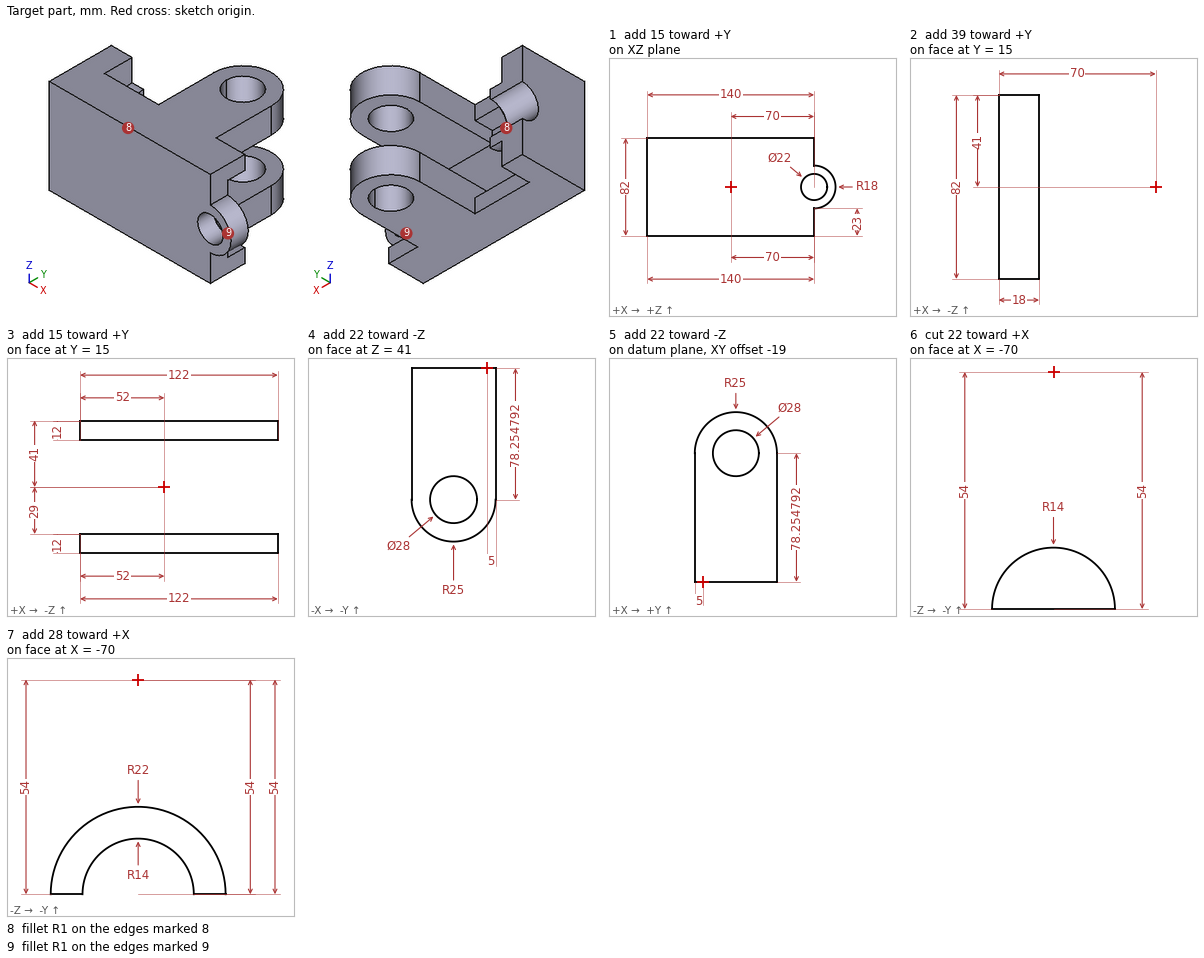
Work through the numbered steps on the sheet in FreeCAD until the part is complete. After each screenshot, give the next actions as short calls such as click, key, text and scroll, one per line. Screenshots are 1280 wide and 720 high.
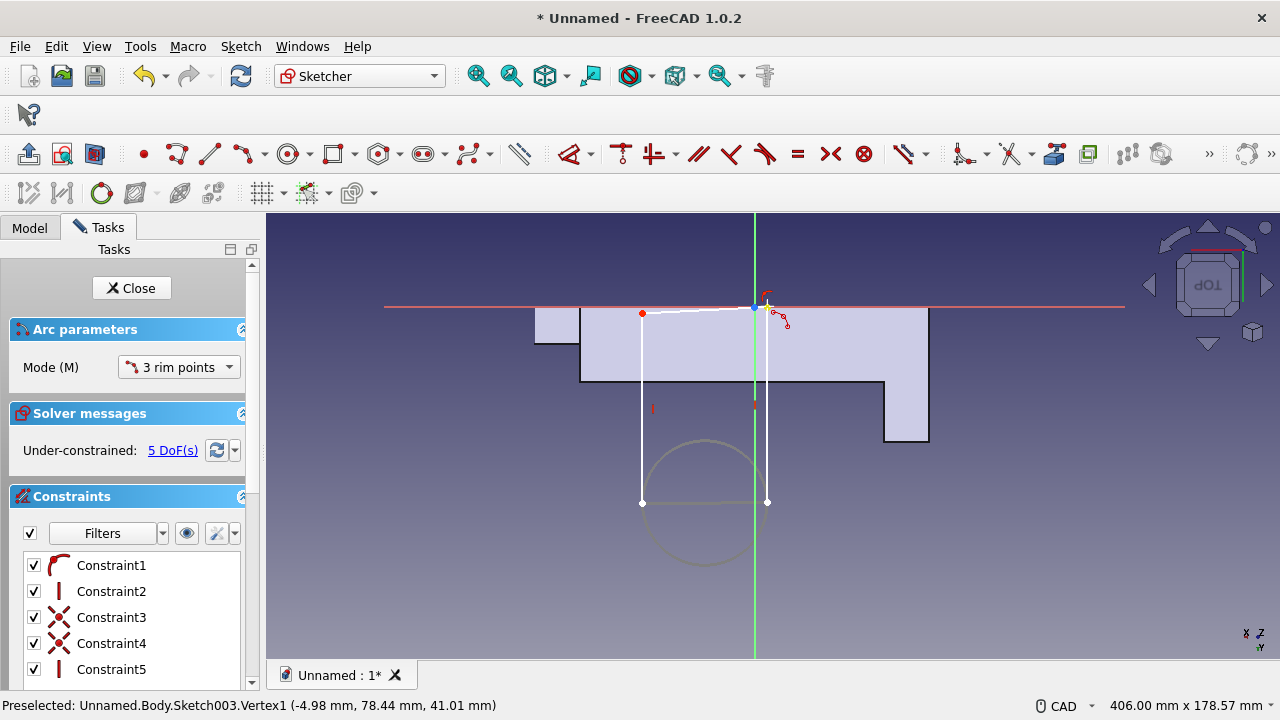
click(705, 565)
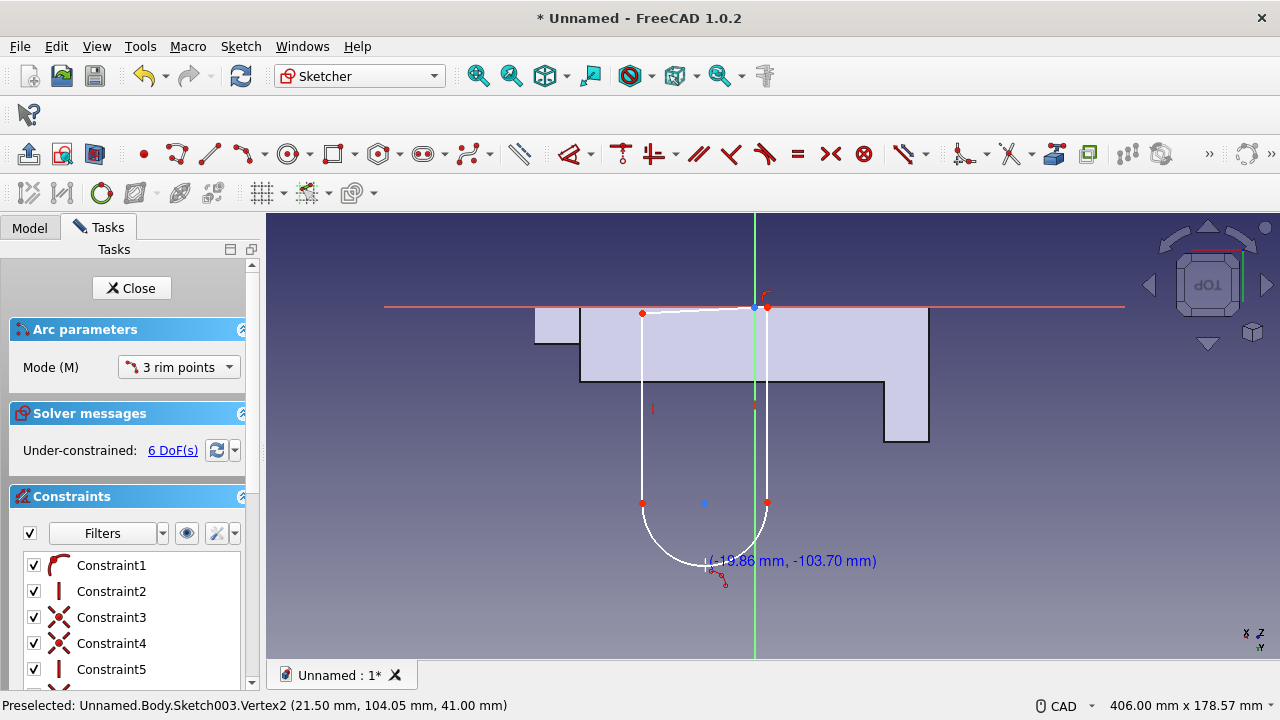
click(288, 154)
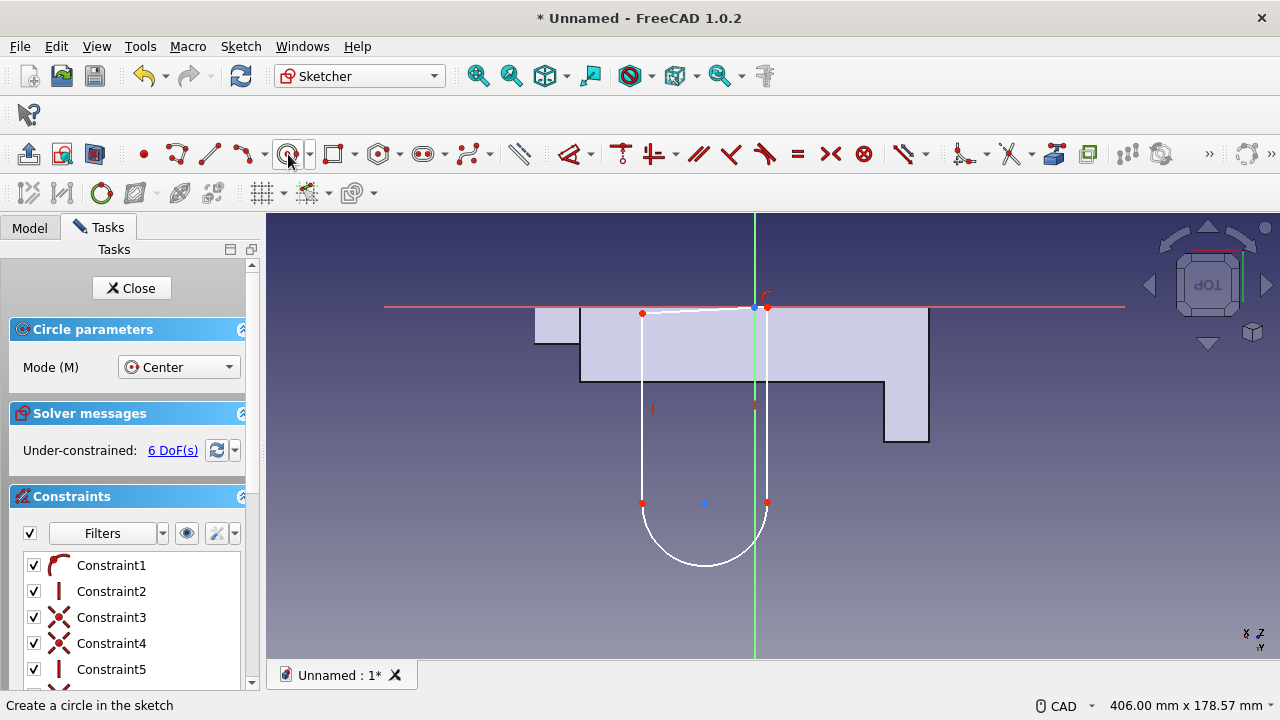
click(705, 502)
click(729, 478)
key(Escape)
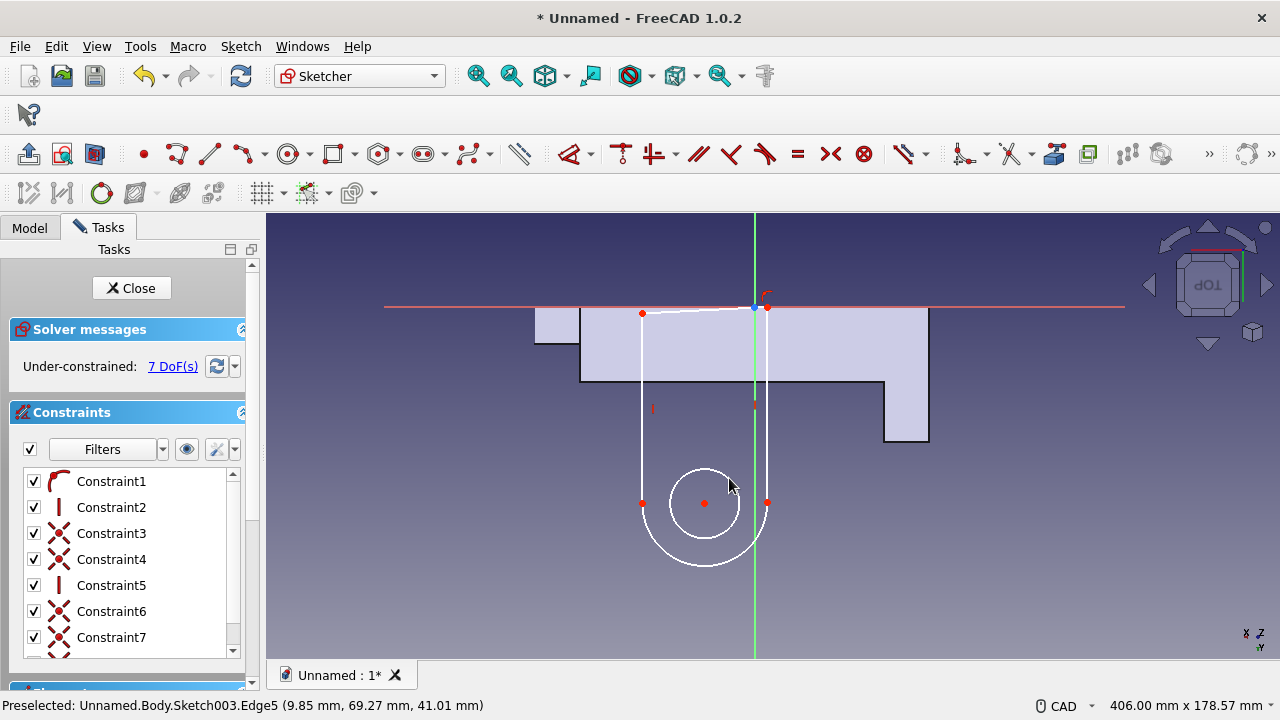
click(767, 444)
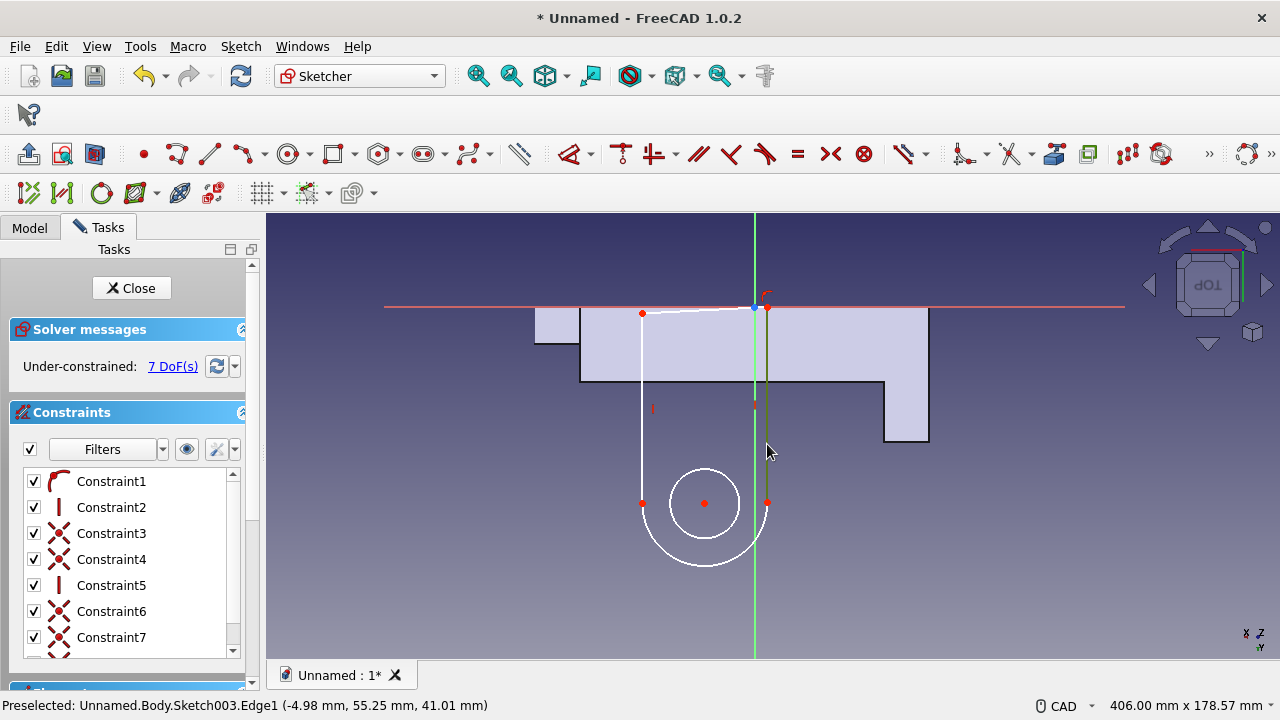
click(668, 554)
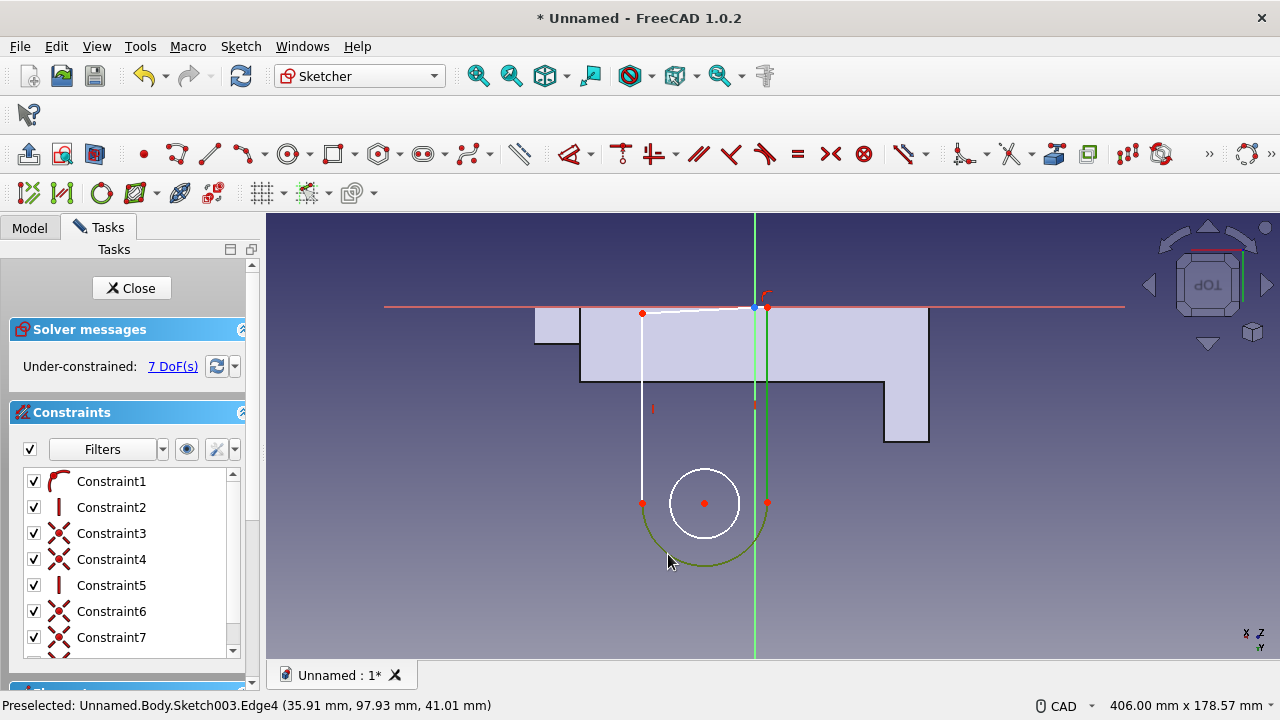
click(765, 154)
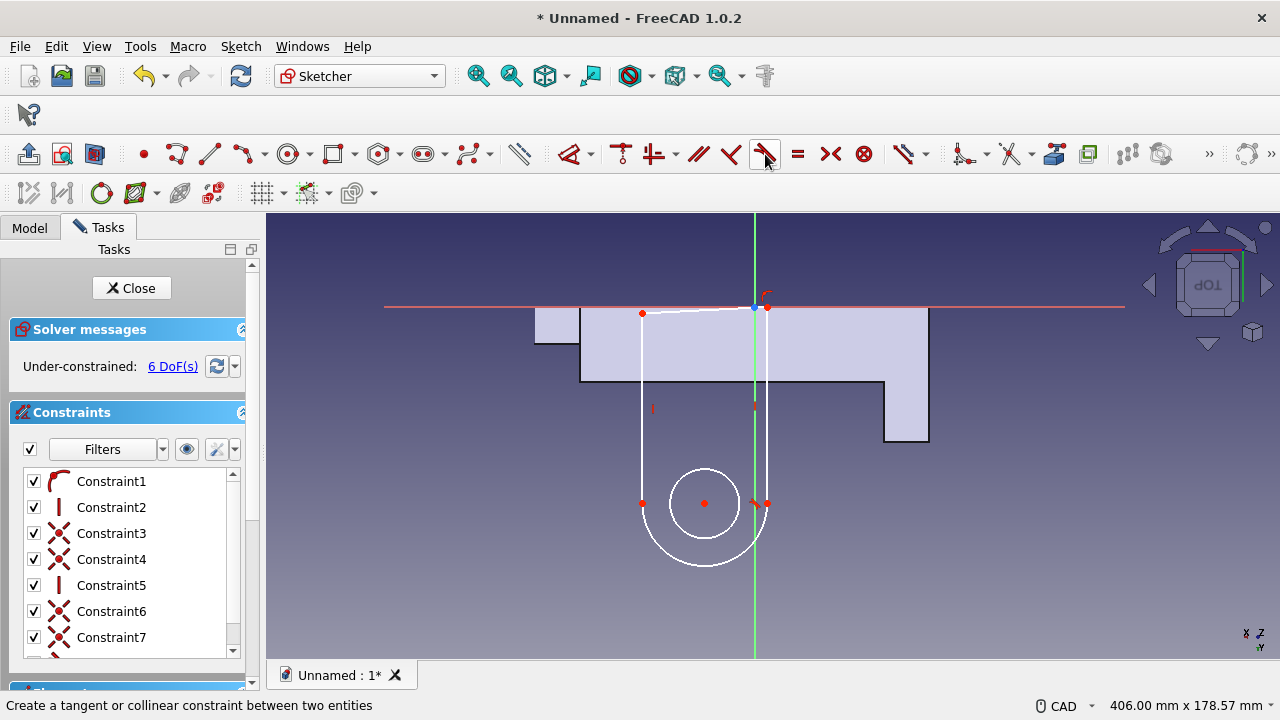
click(642, 370)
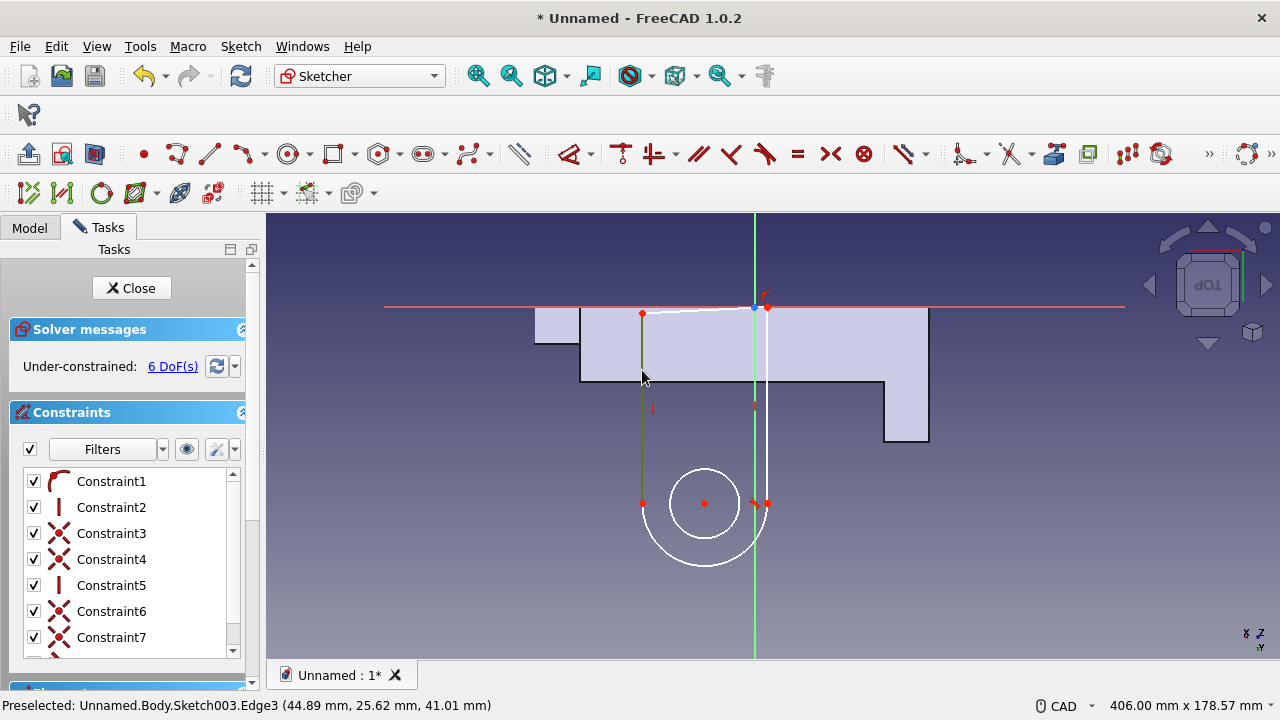
click(668, 554)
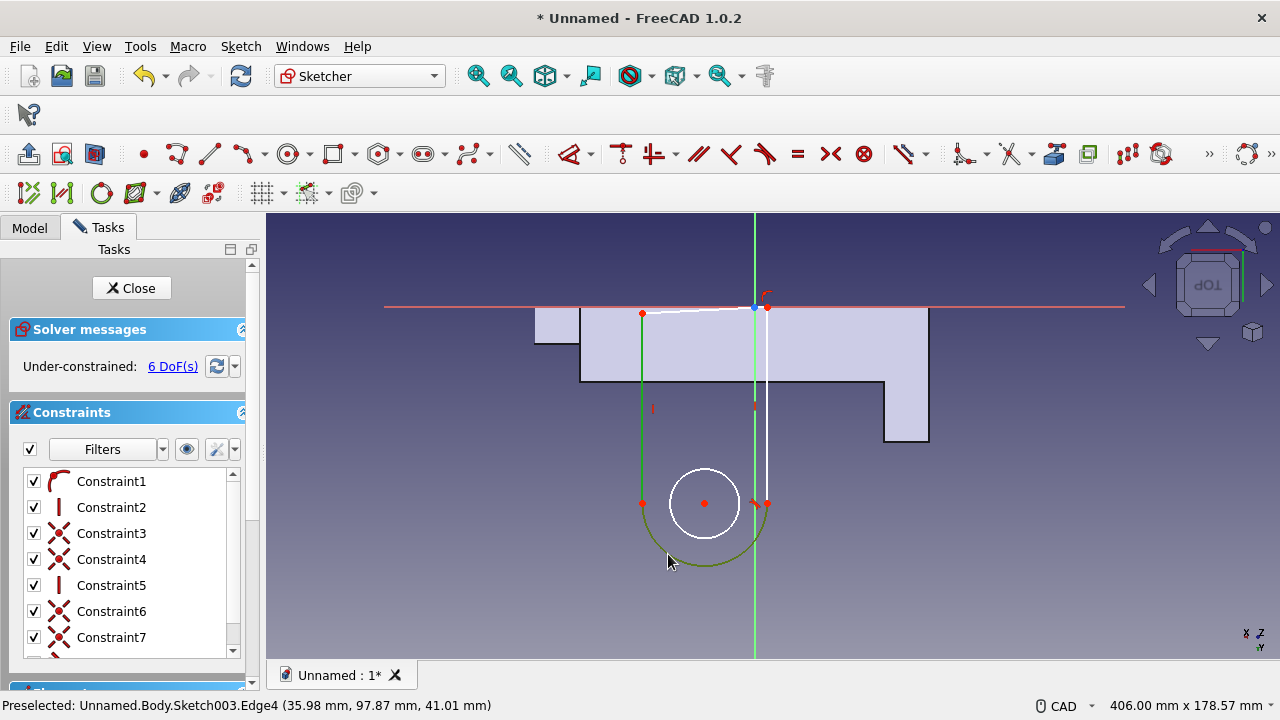
click(765, 154)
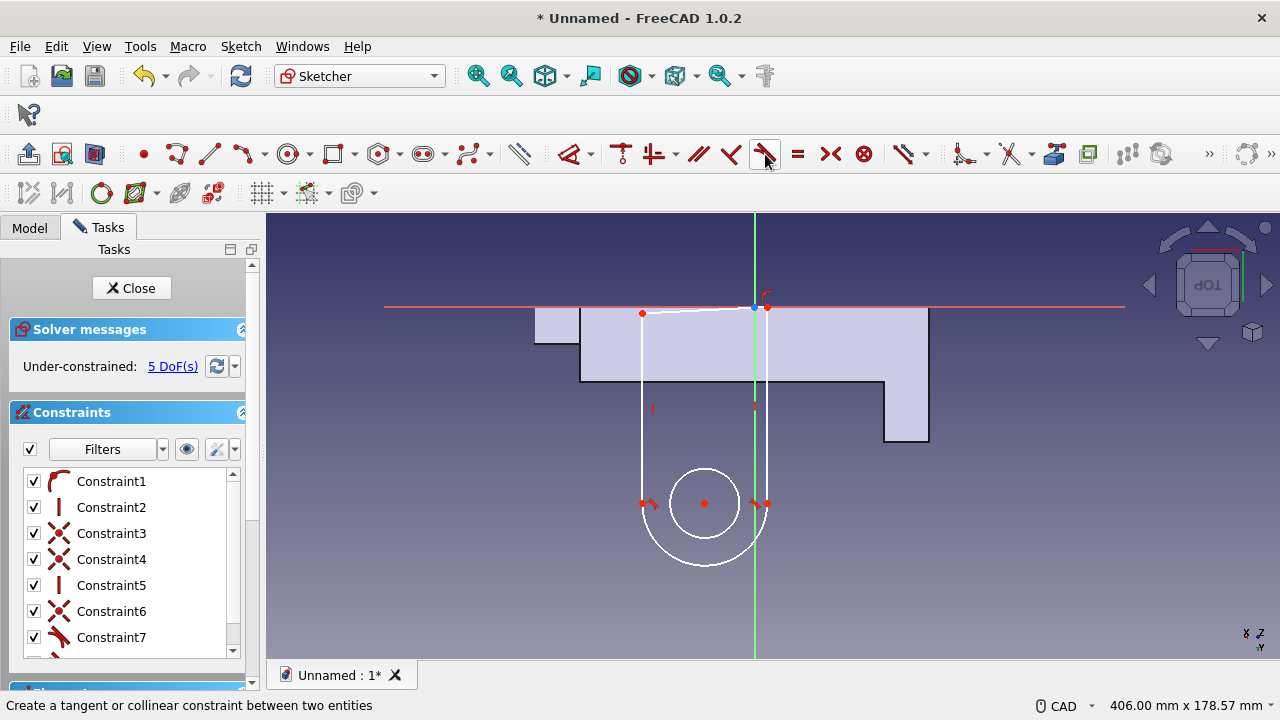
click(730, 309)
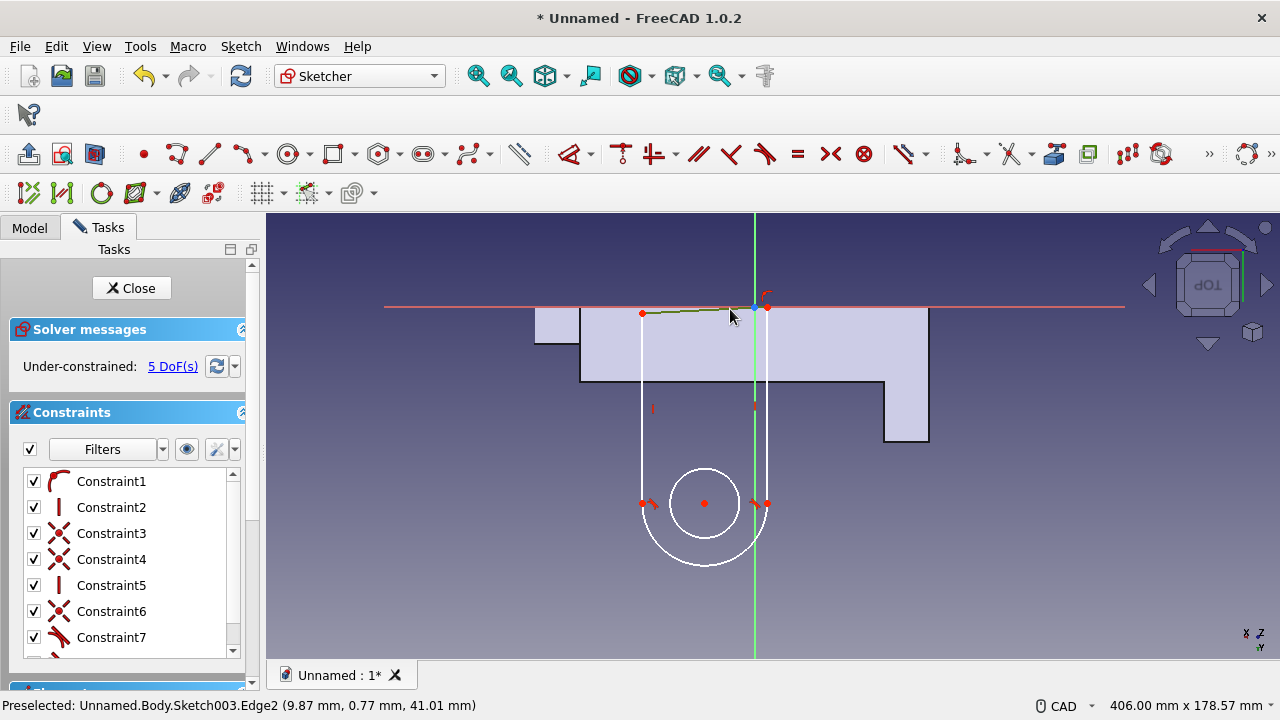
click(676, 154)